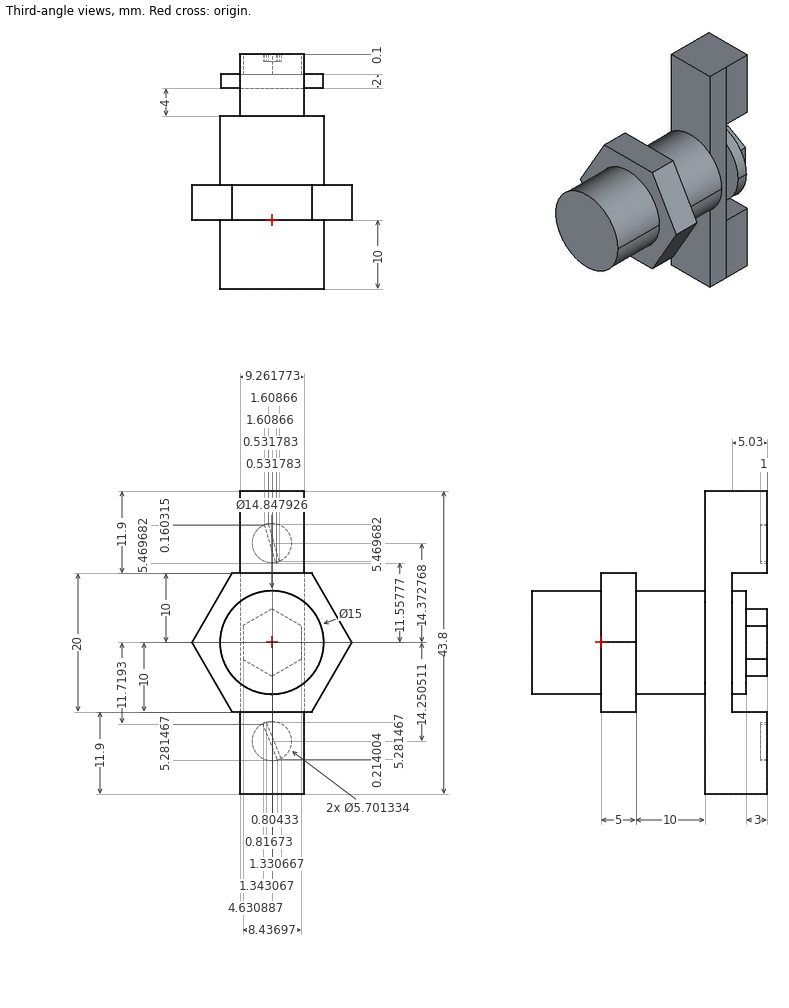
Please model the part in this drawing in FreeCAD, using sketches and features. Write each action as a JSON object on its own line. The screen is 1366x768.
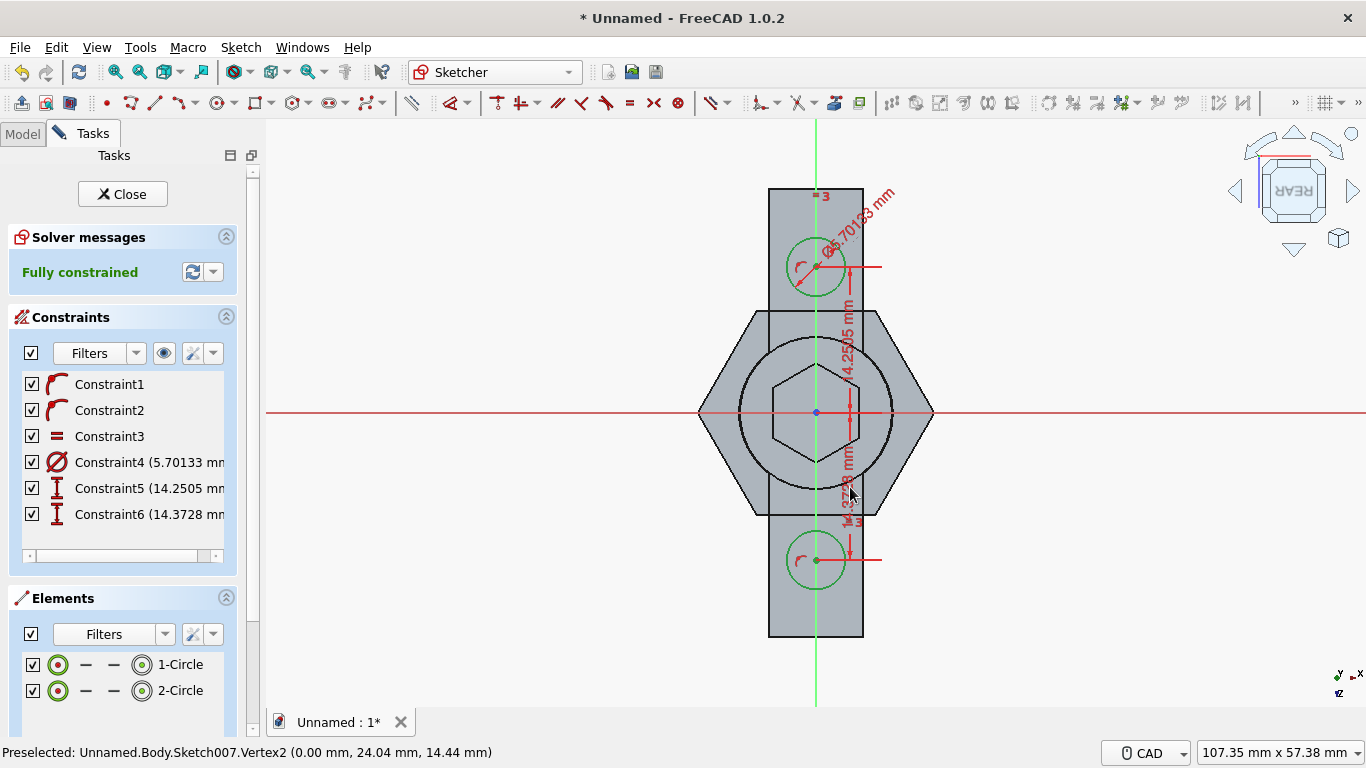
{"action": "left_click", "coordinate": [123, 194]}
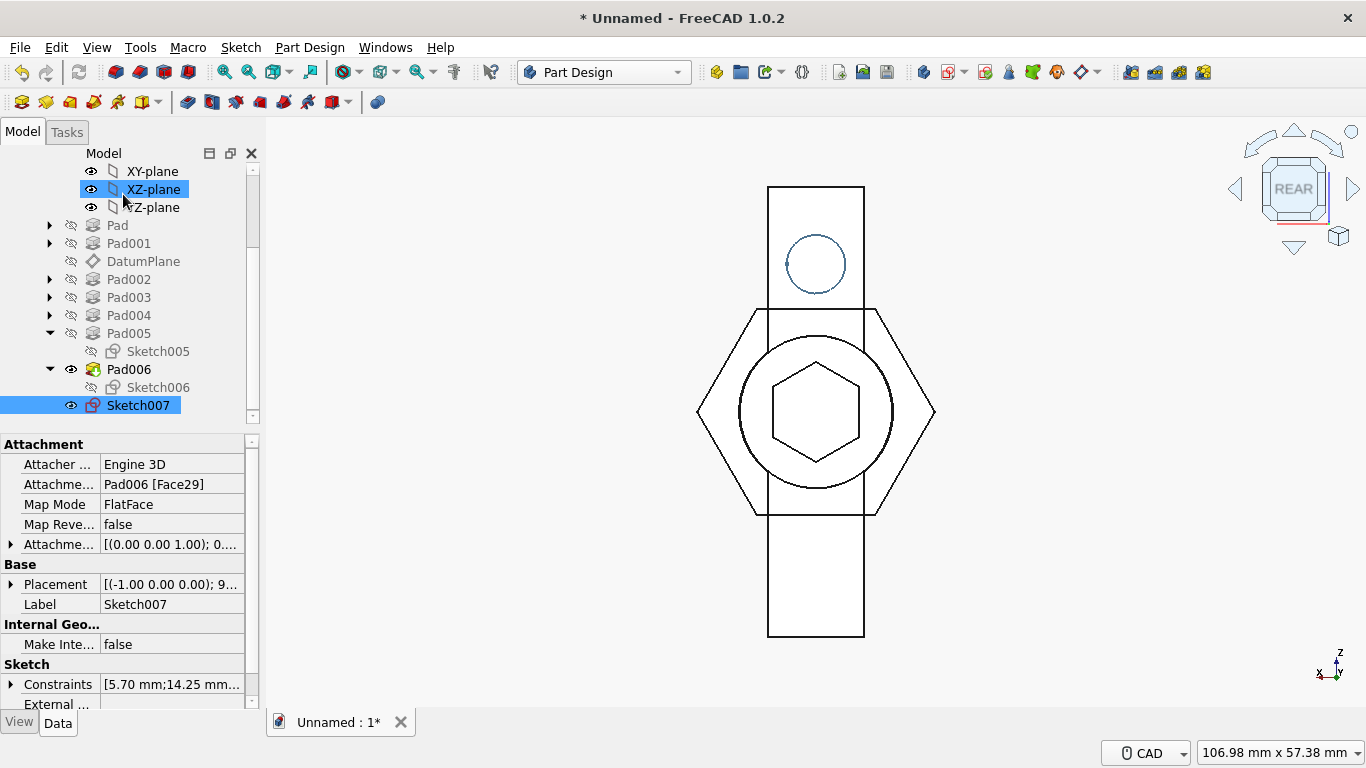
{"action": "left_click", "coordinate": [188, 102]}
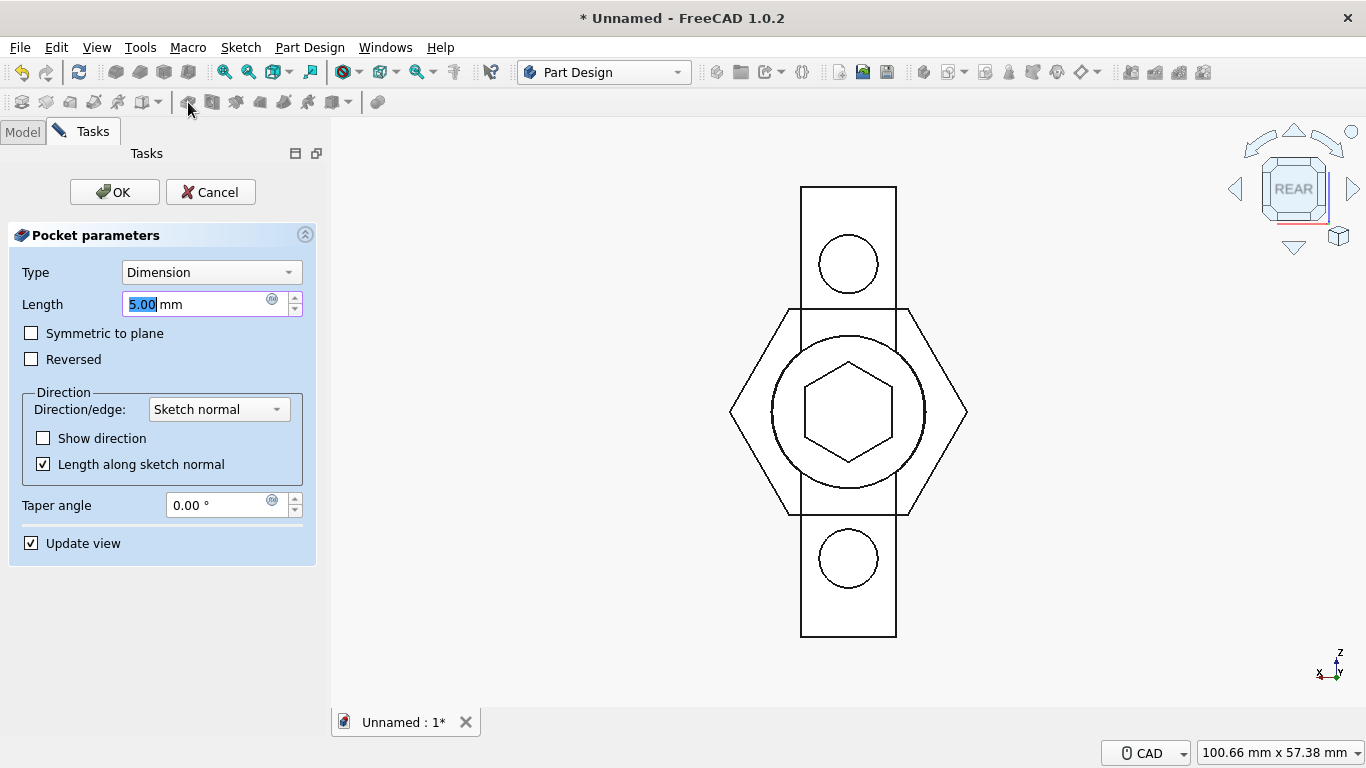
{"action": "type", "text": "0.1"}
{"action": "key", "text": "Tab"}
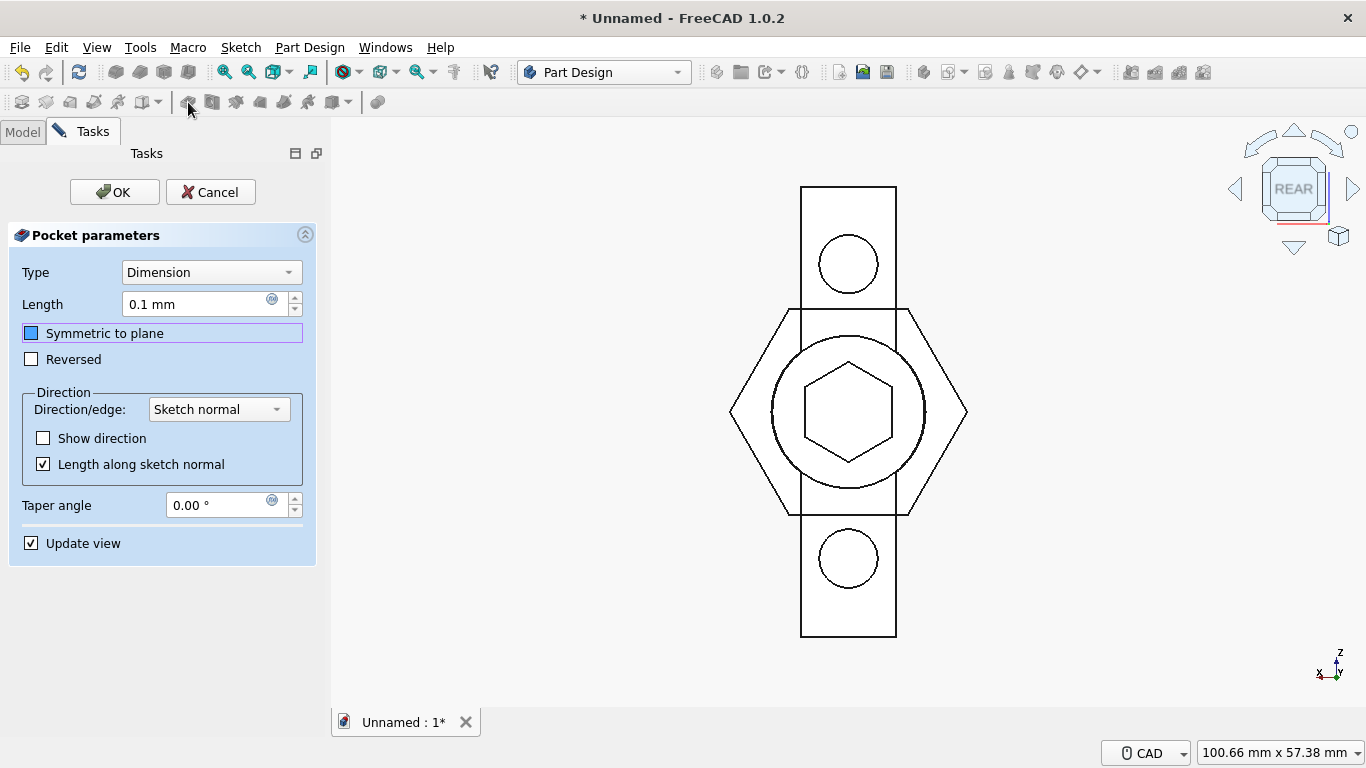
{"action": "left_click", "coordinate": [115, 192]}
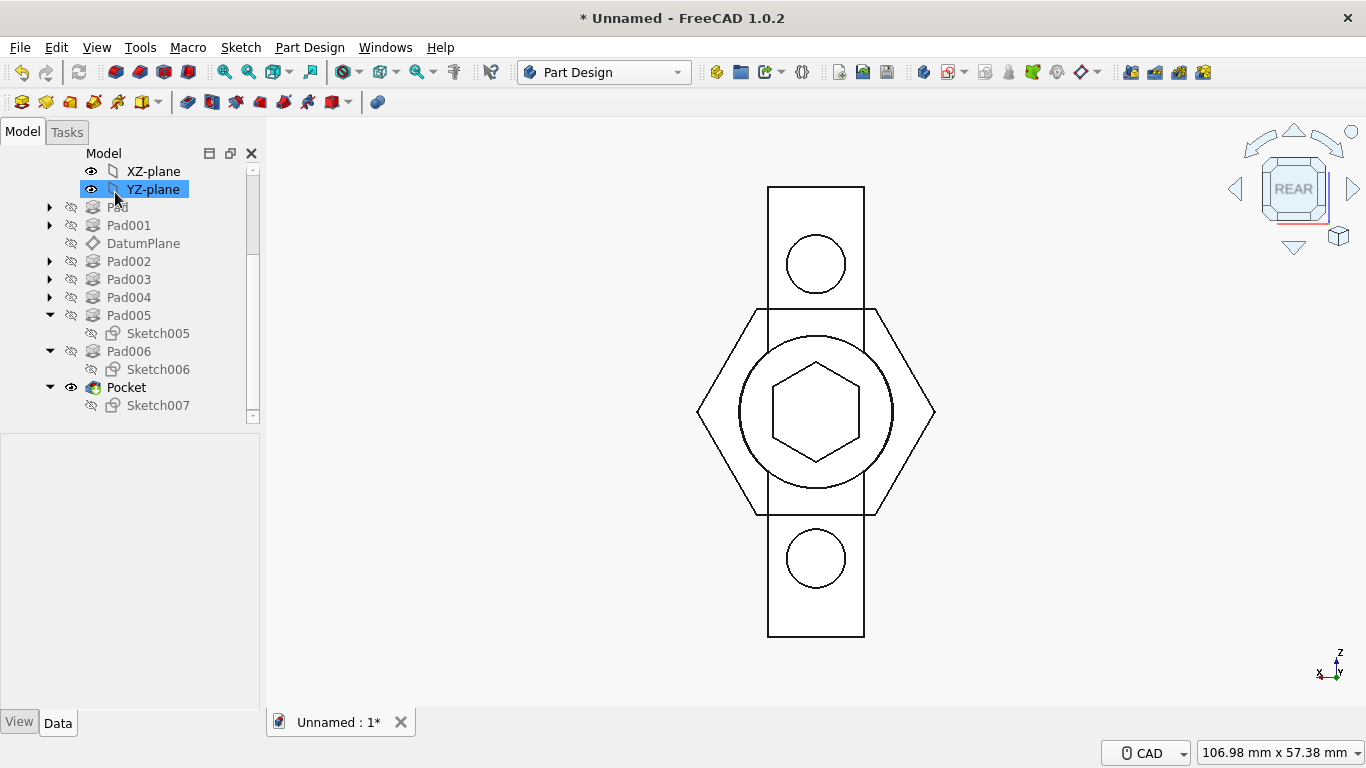
{"action": "left_click", "coordinate": [816, 558]}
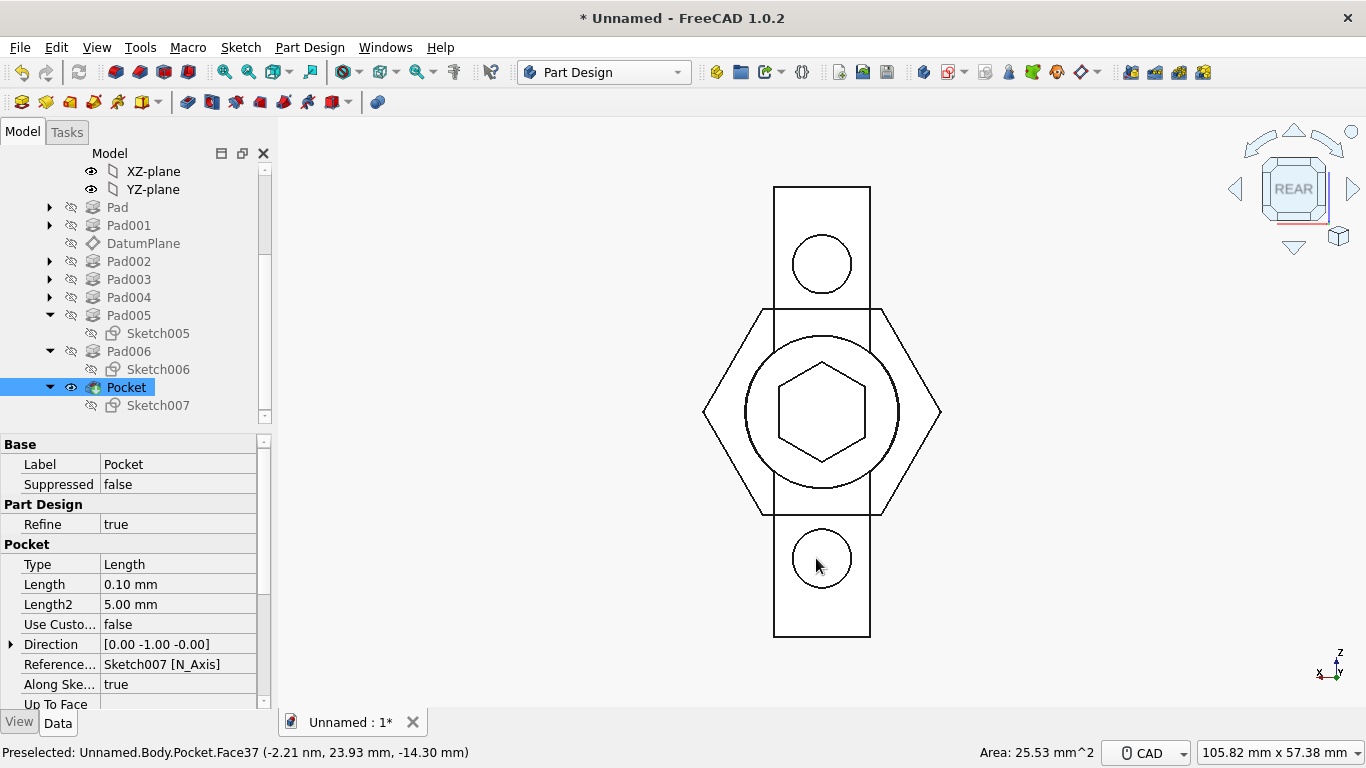
{"action": "left_click", "coordinate": [948, 72]}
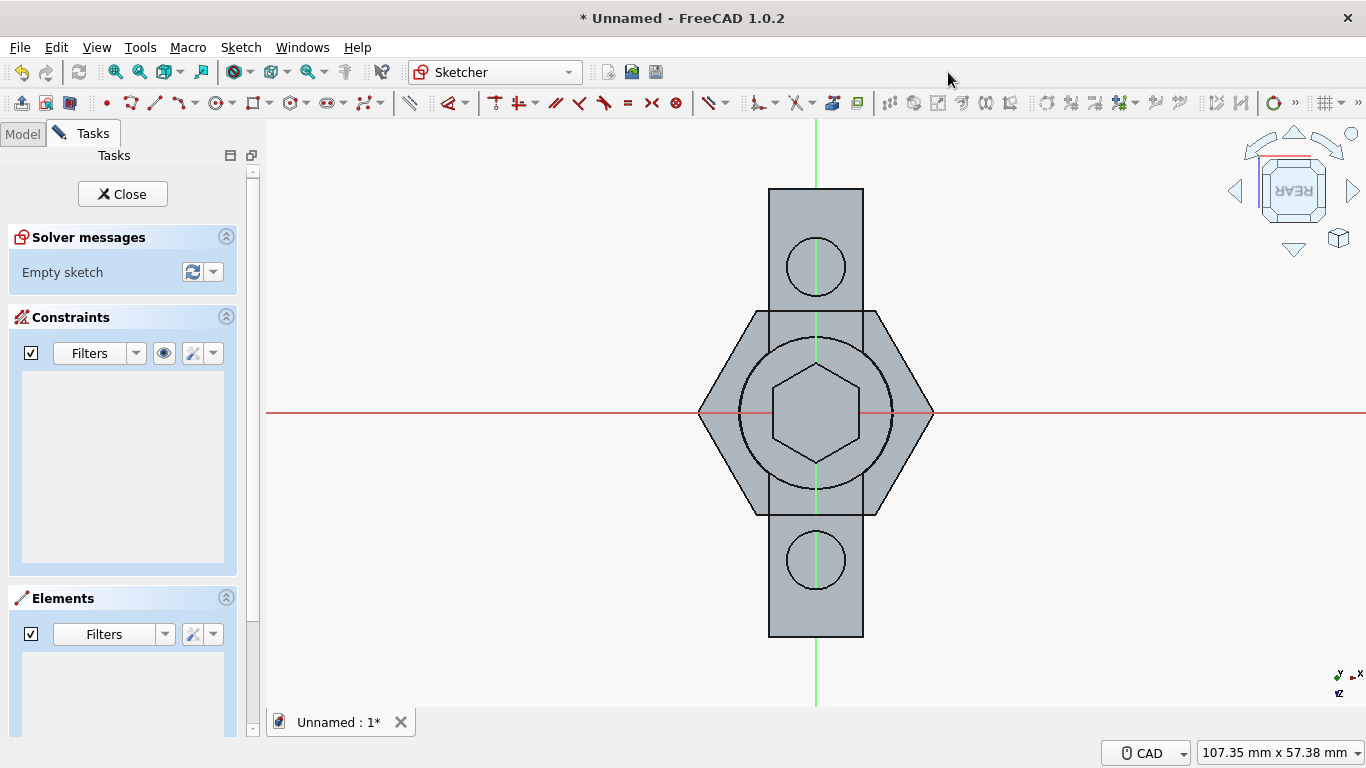
{"action": "left_click", "coordinate": [132, 104]}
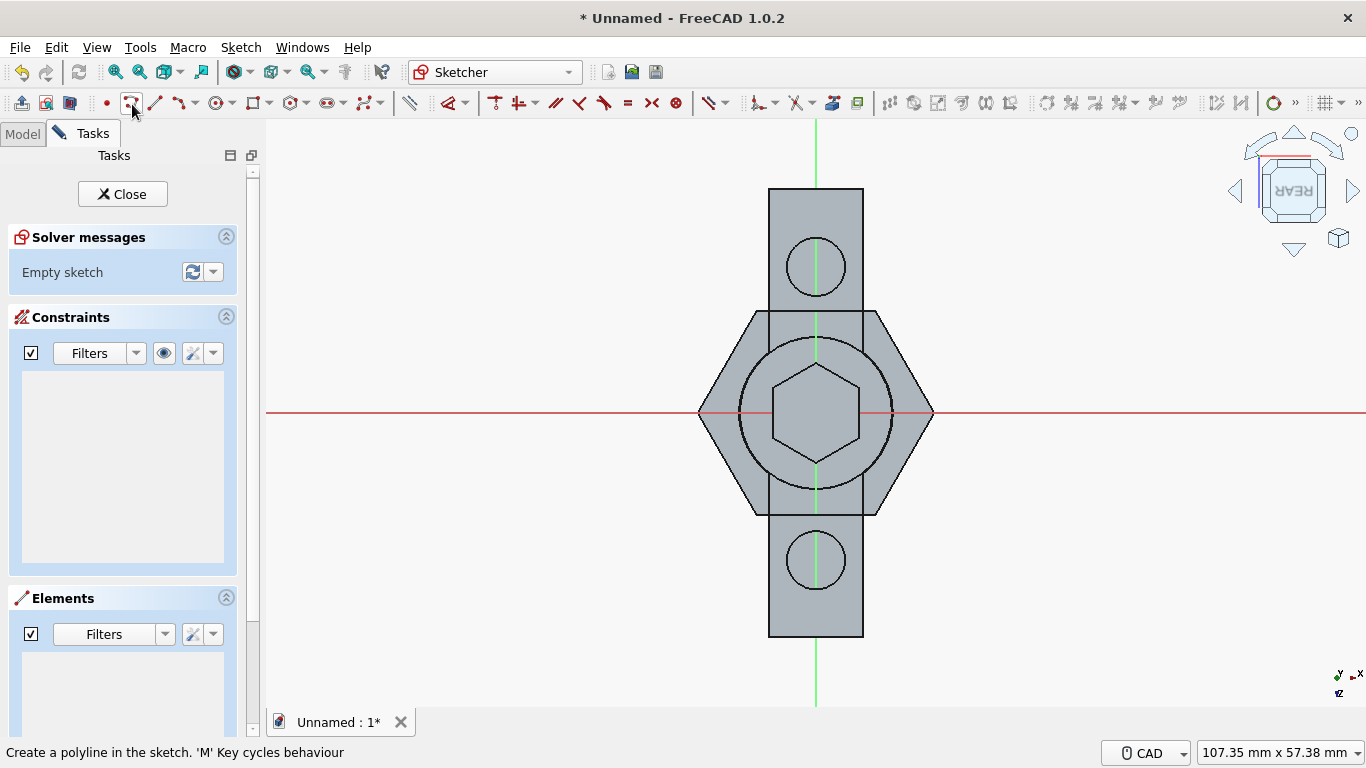
{"action": "scroll", "coordinate": [808, 295], "scroll_direction": "up", "scroll_amount": 4}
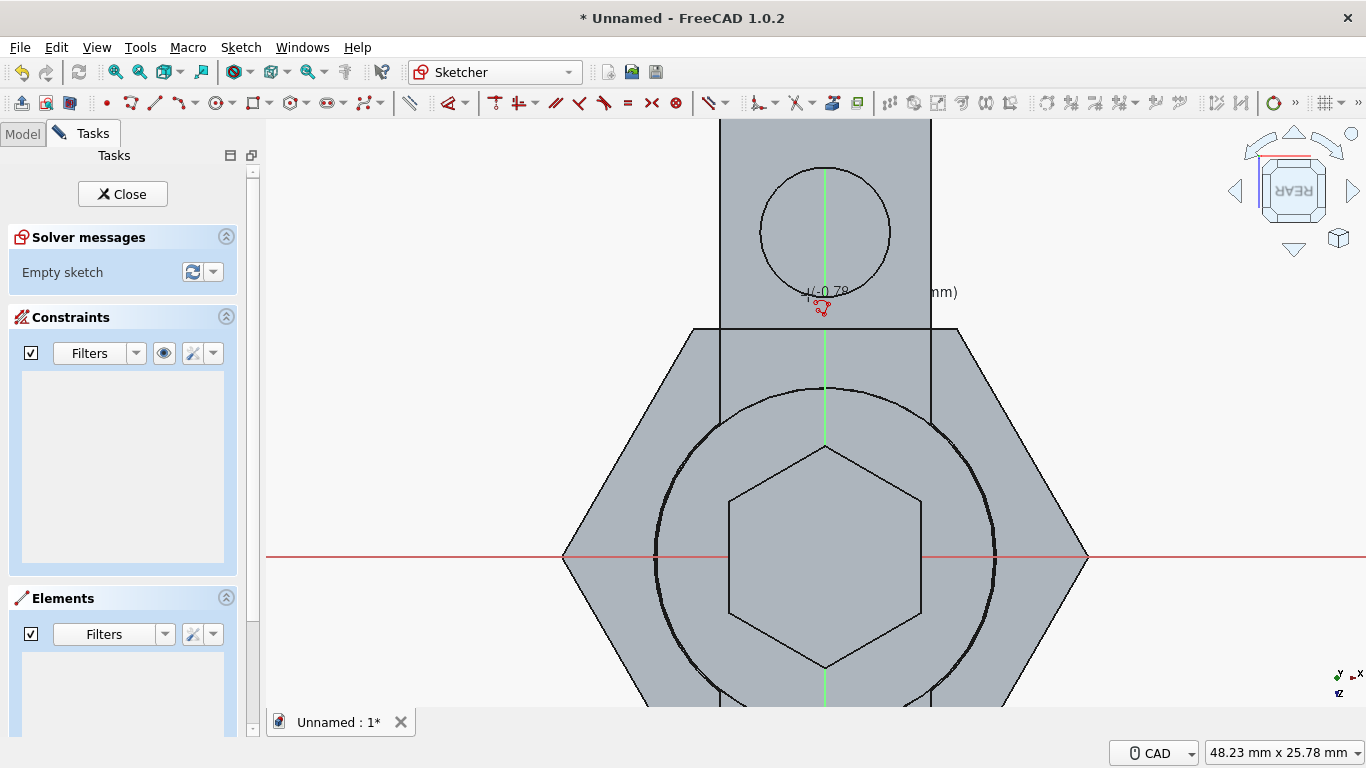
{"action": "left_click", "coordinate": [807, 295]}
{"action": "left_click", "coordinate": [856, 174]}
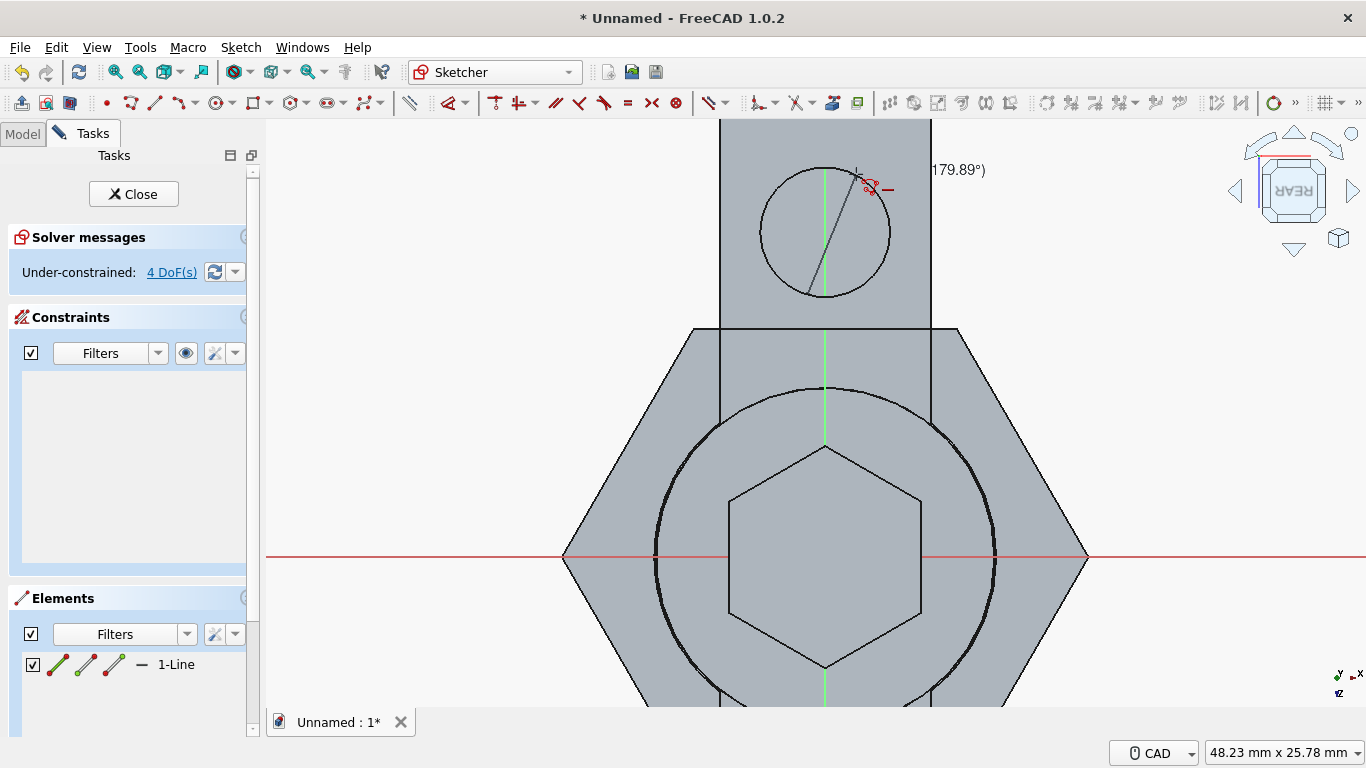
{"action": "scroll", "coordinate": [844, 170], "scroll_direction": "up", "scroll_amount": 2}